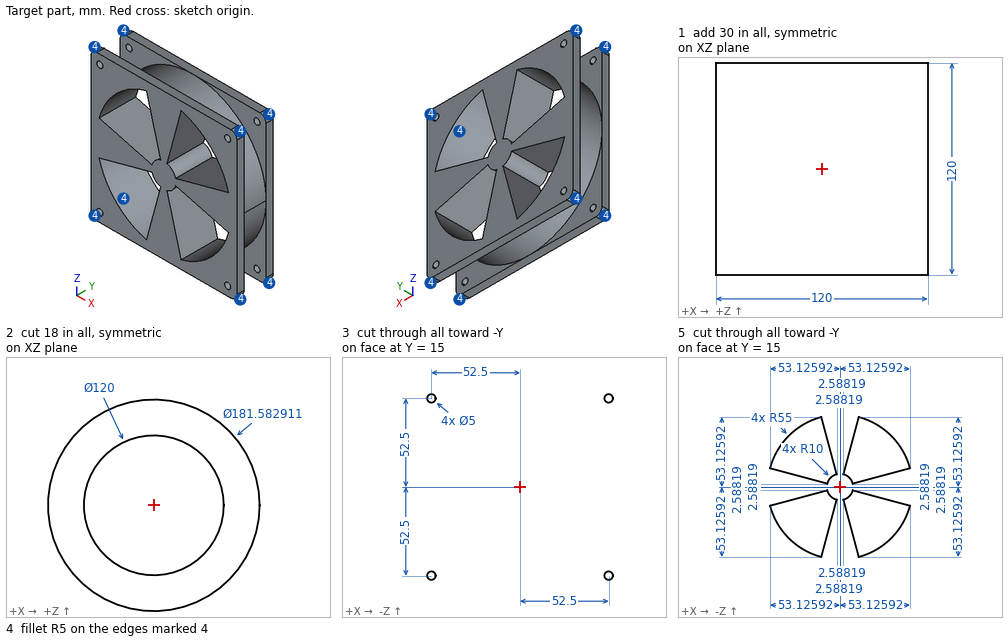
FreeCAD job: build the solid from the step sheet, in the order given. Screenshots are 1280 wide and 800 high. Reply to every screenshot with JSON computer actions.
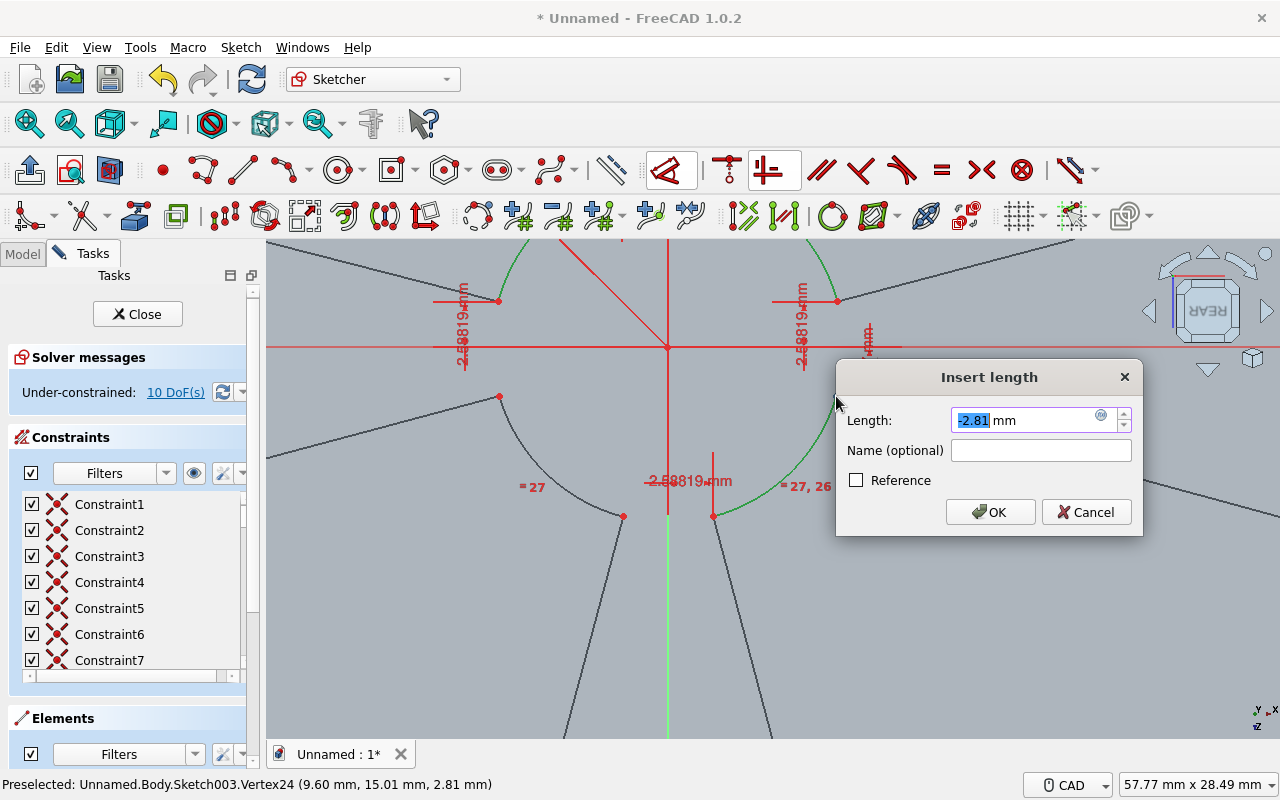
{"action": "type", "text": "-2.58819"}
{"action": "key", "text": "Return"}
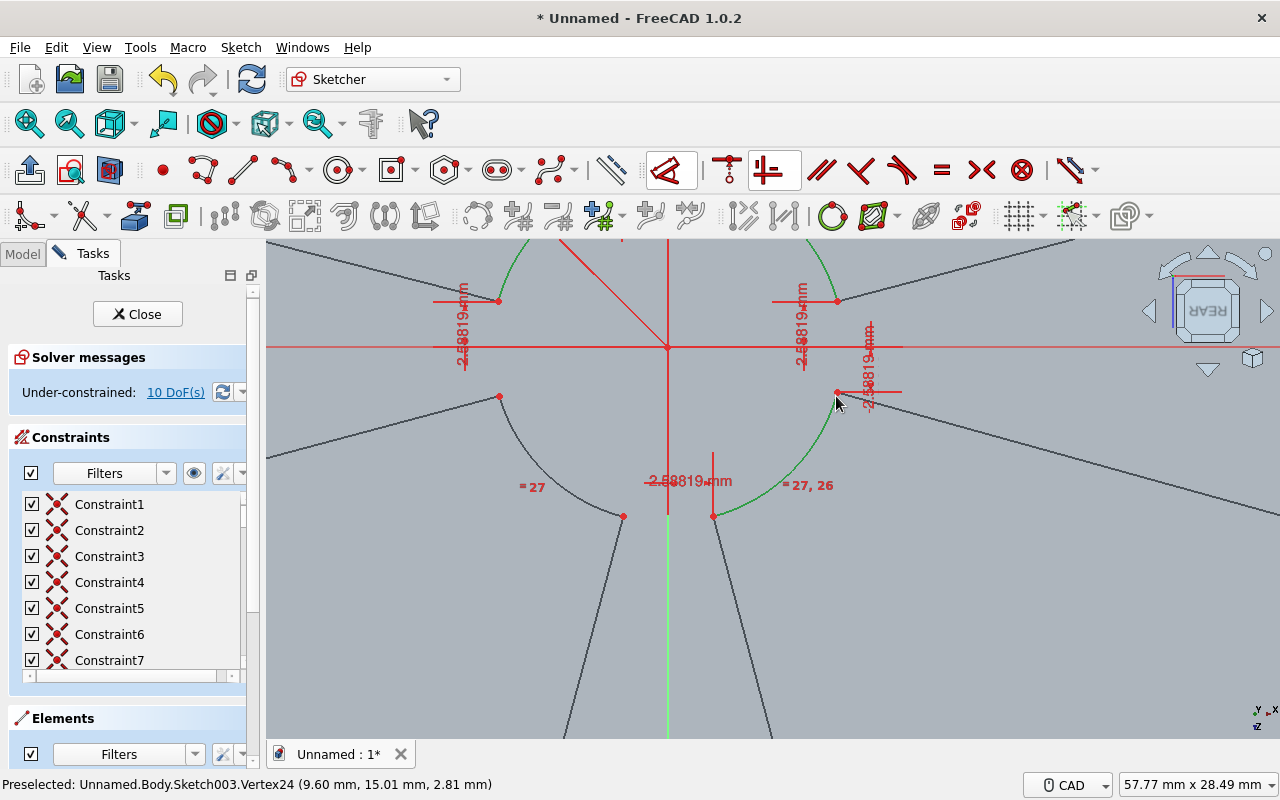
{"action": "left_click", "coordinate": [623, 517]}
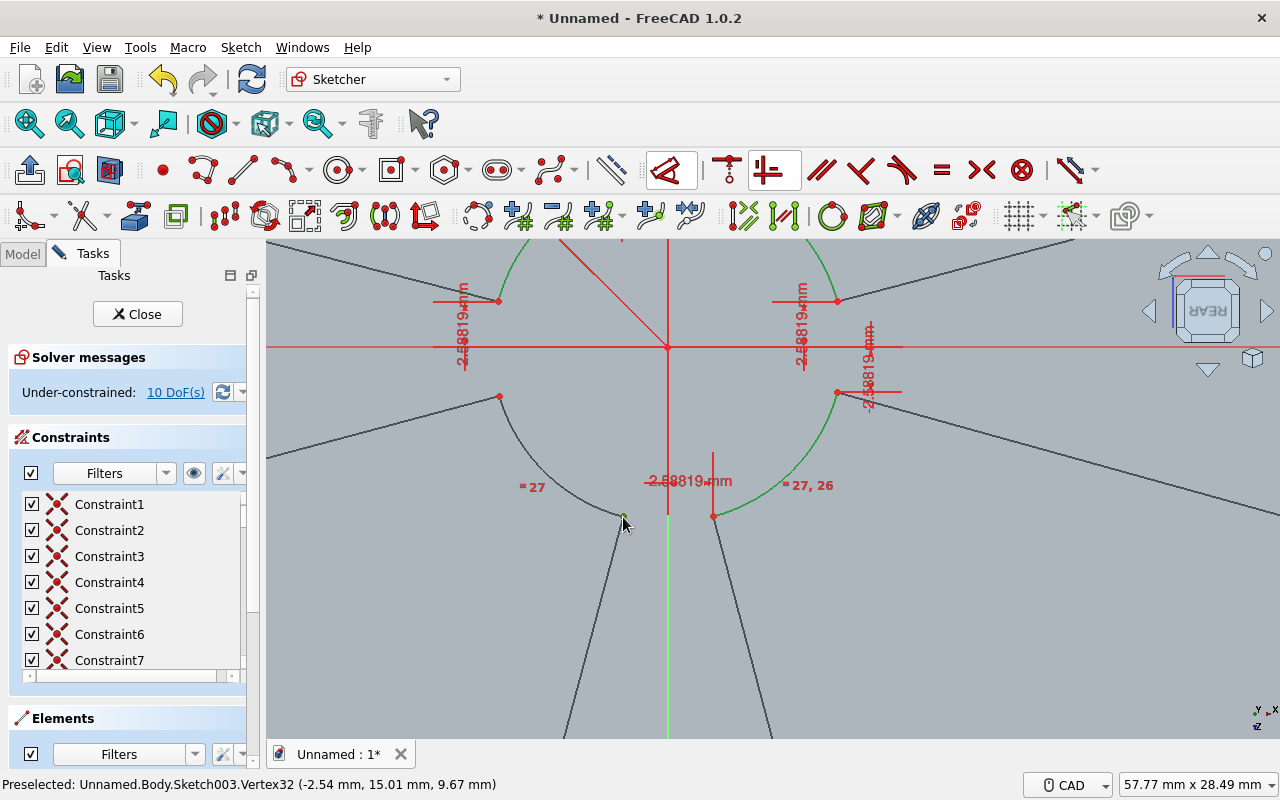
{"action": "key", "text": "l"}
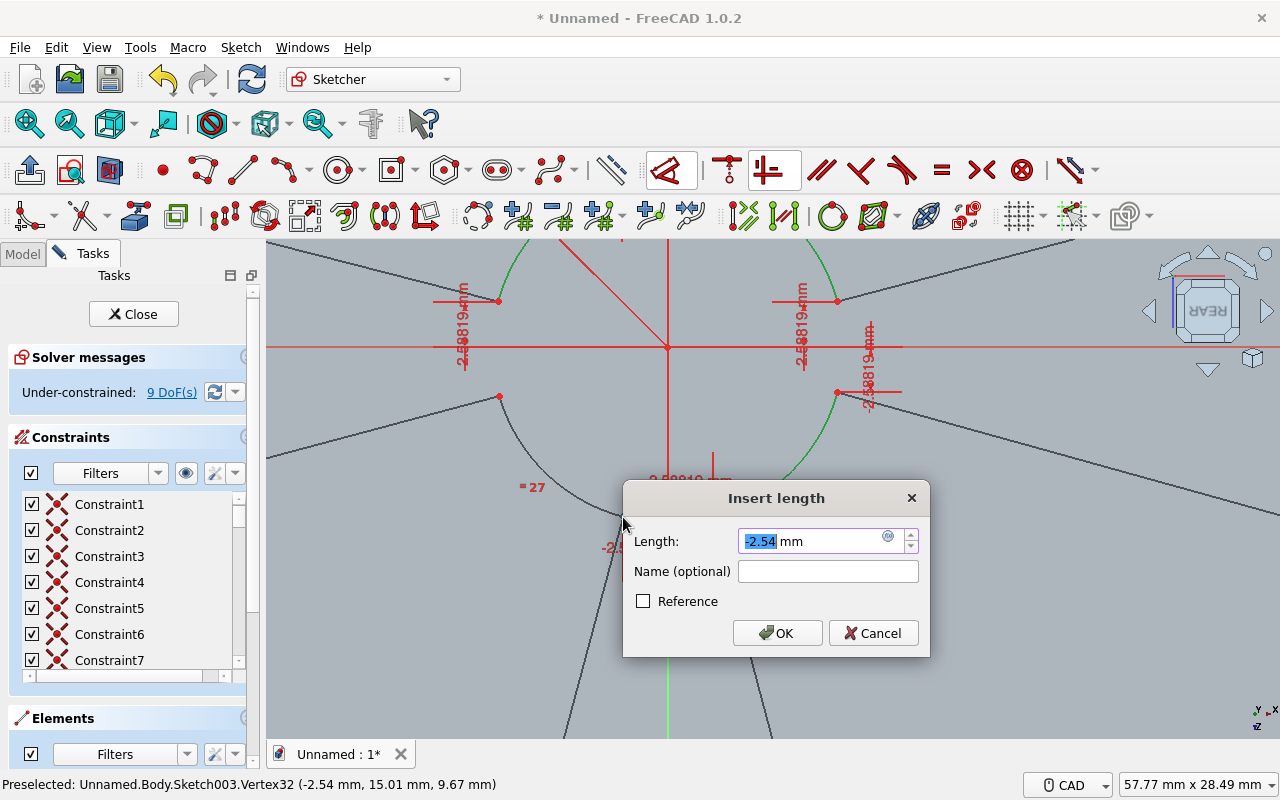
{"action": "type", "text": "-2.58819"}
{"action": "key", "text": "Return"}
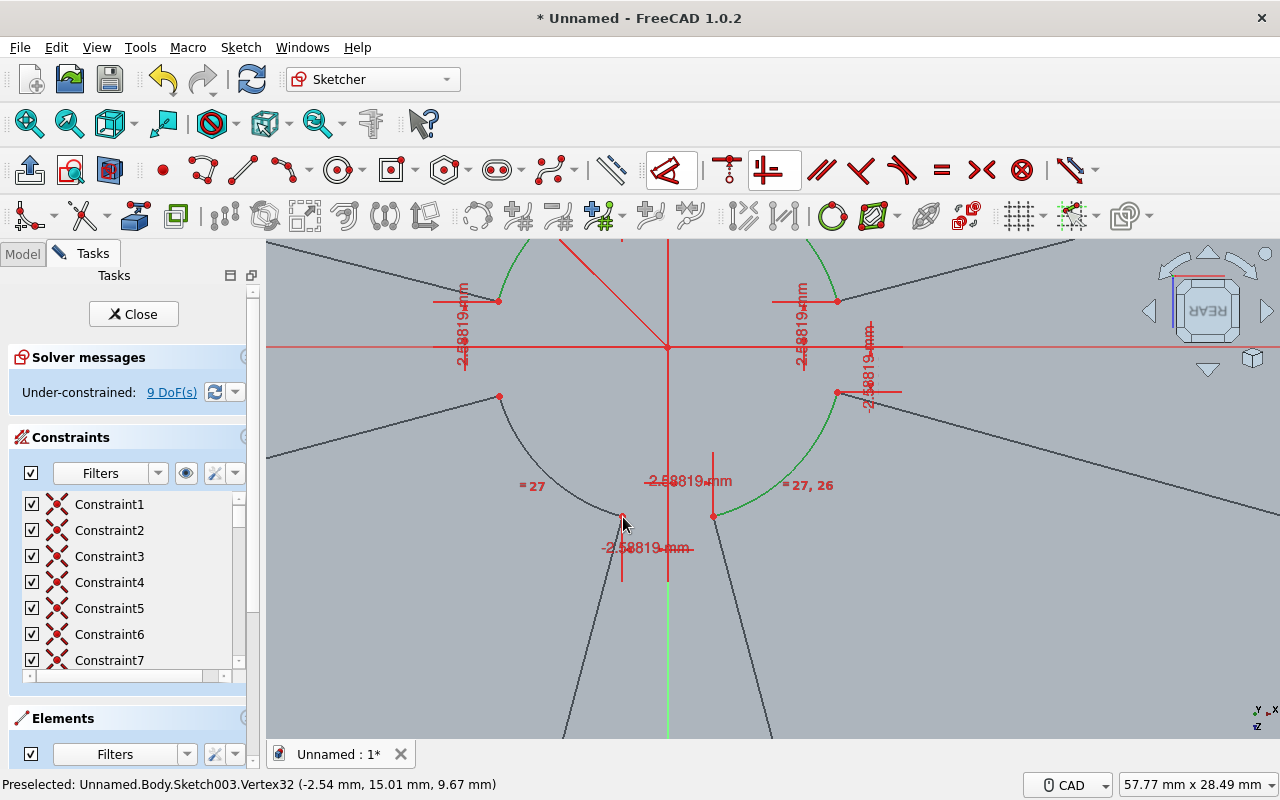
{"action": "left_click", "coordinate": [499, 396]}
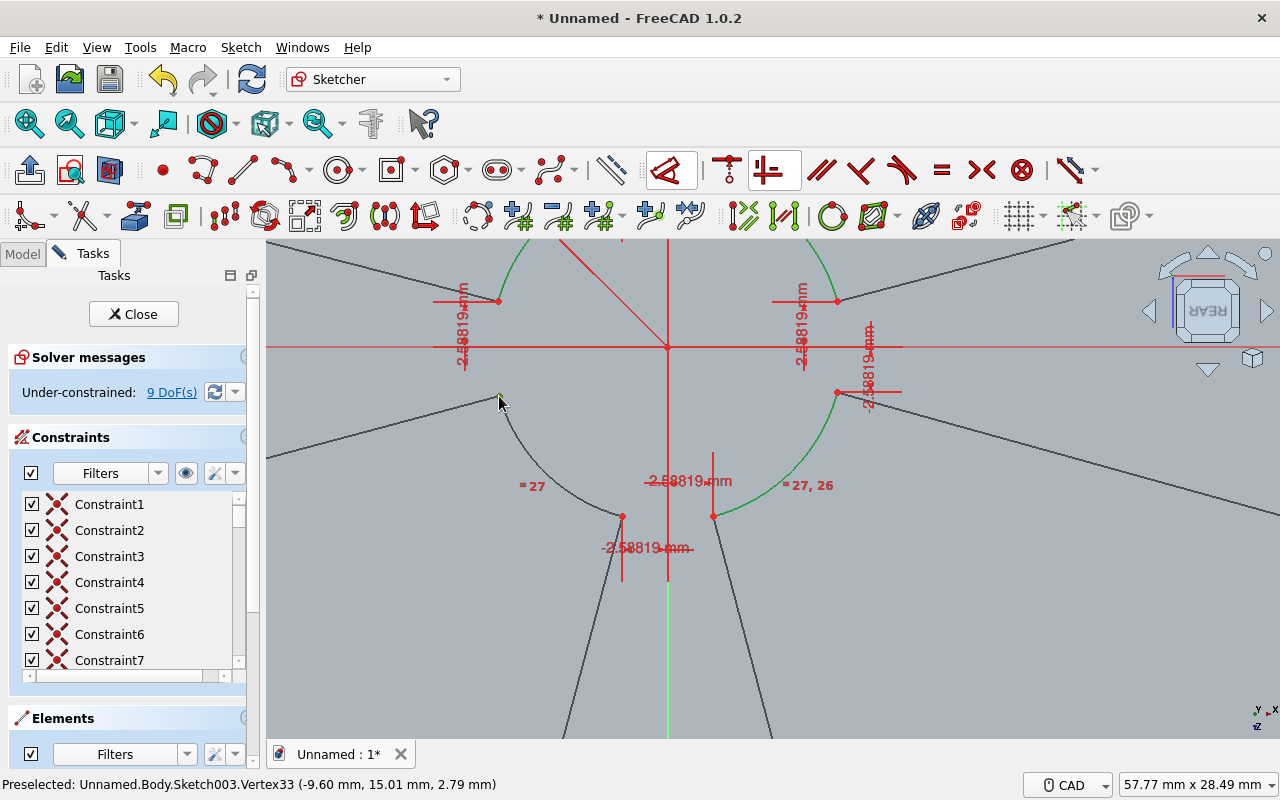
{"action": "left_click", "coordinate": [692, 170]}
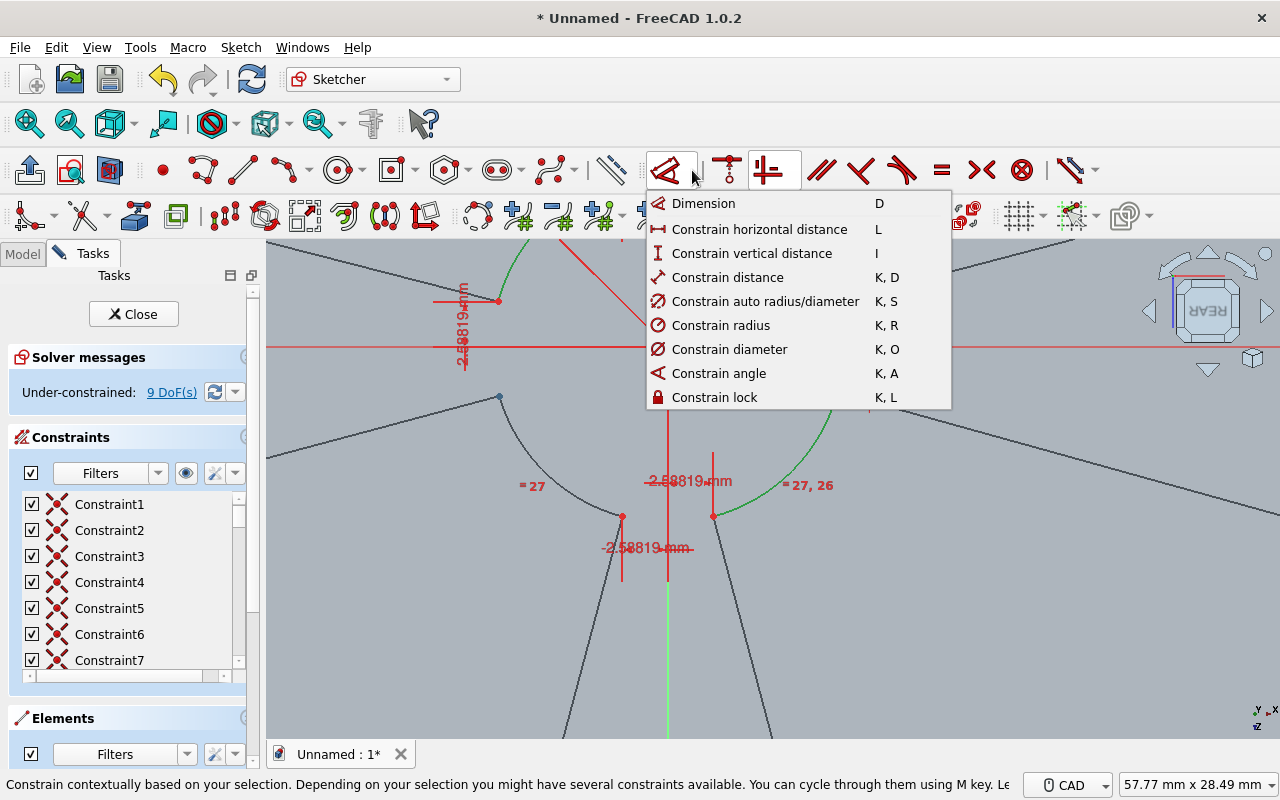
{"action": "left_click", "coordinate": [799, 253]}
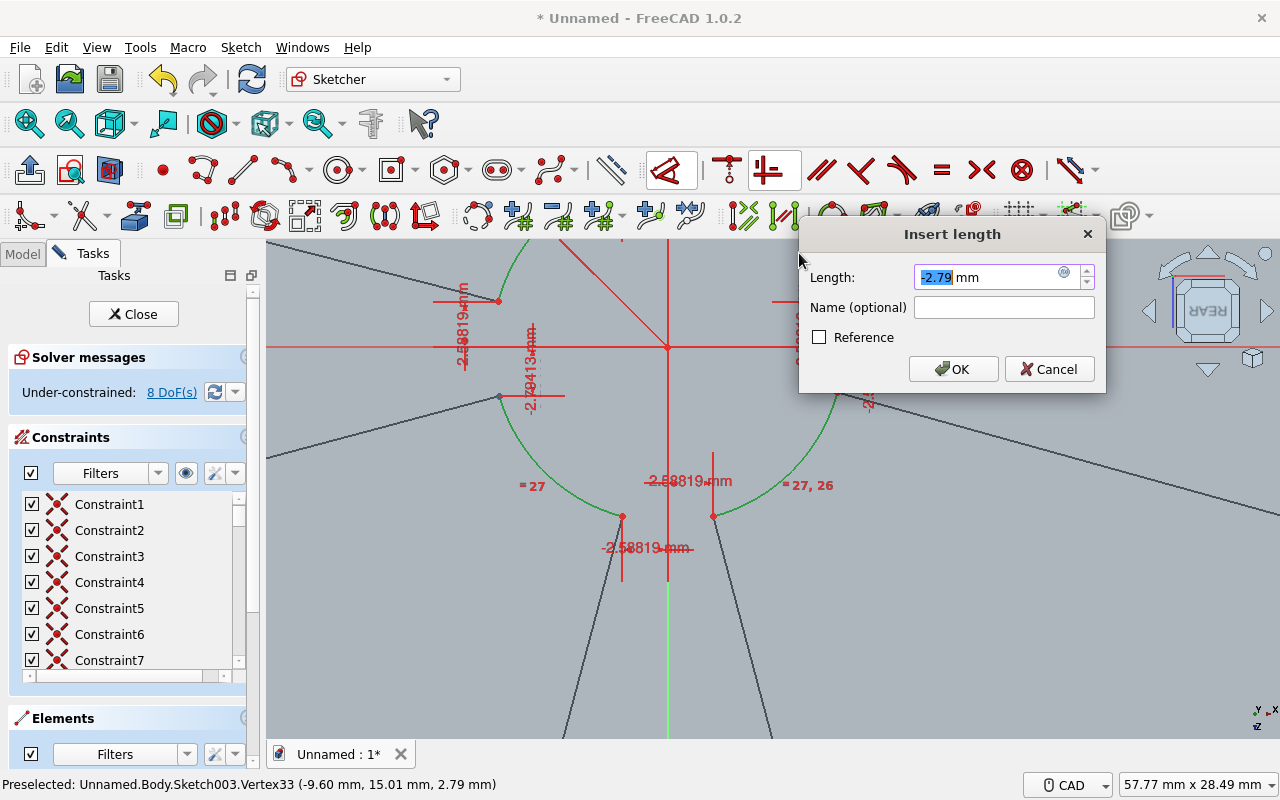
{"action": "type", "text": "-2.58819"}
{"action": "key", "text": "Return"}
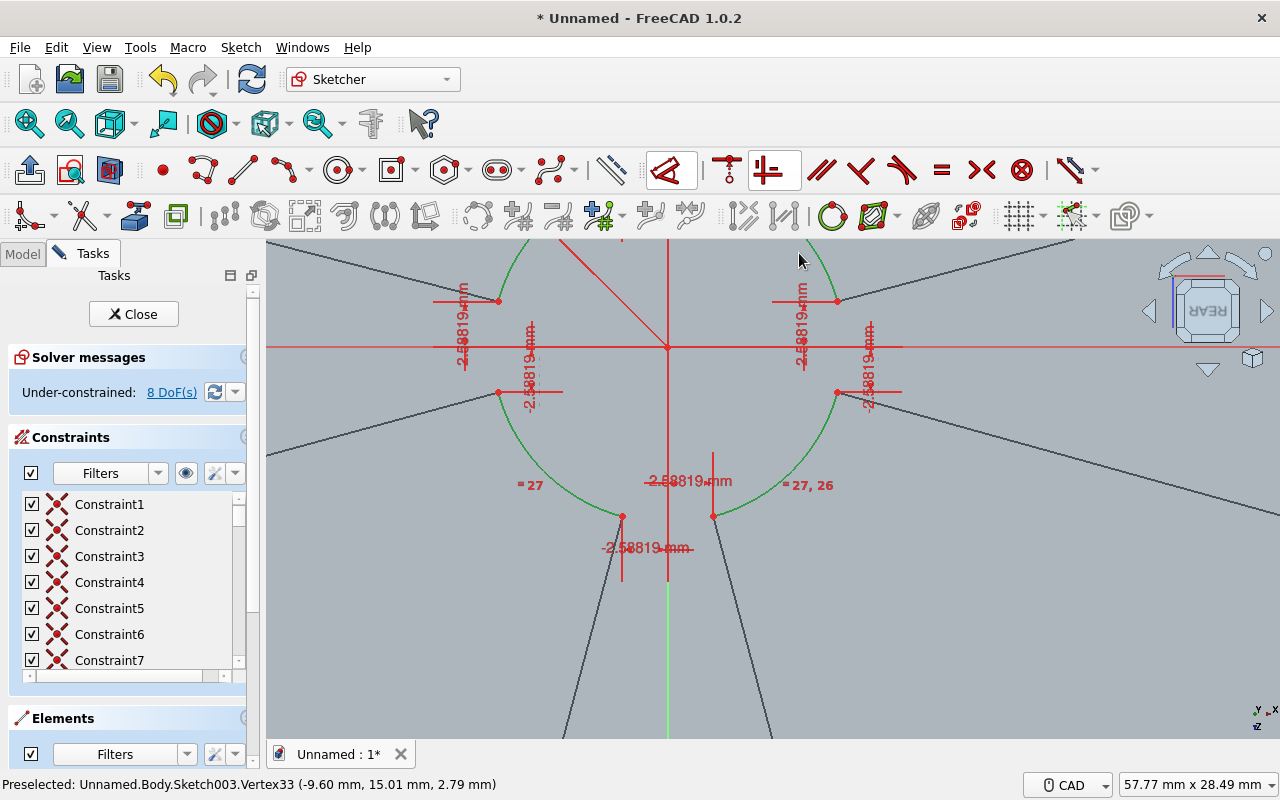
{"action": "scroll", "coordinate": [712, 517], "scroll_direction": "down", "scroll_amount": 9}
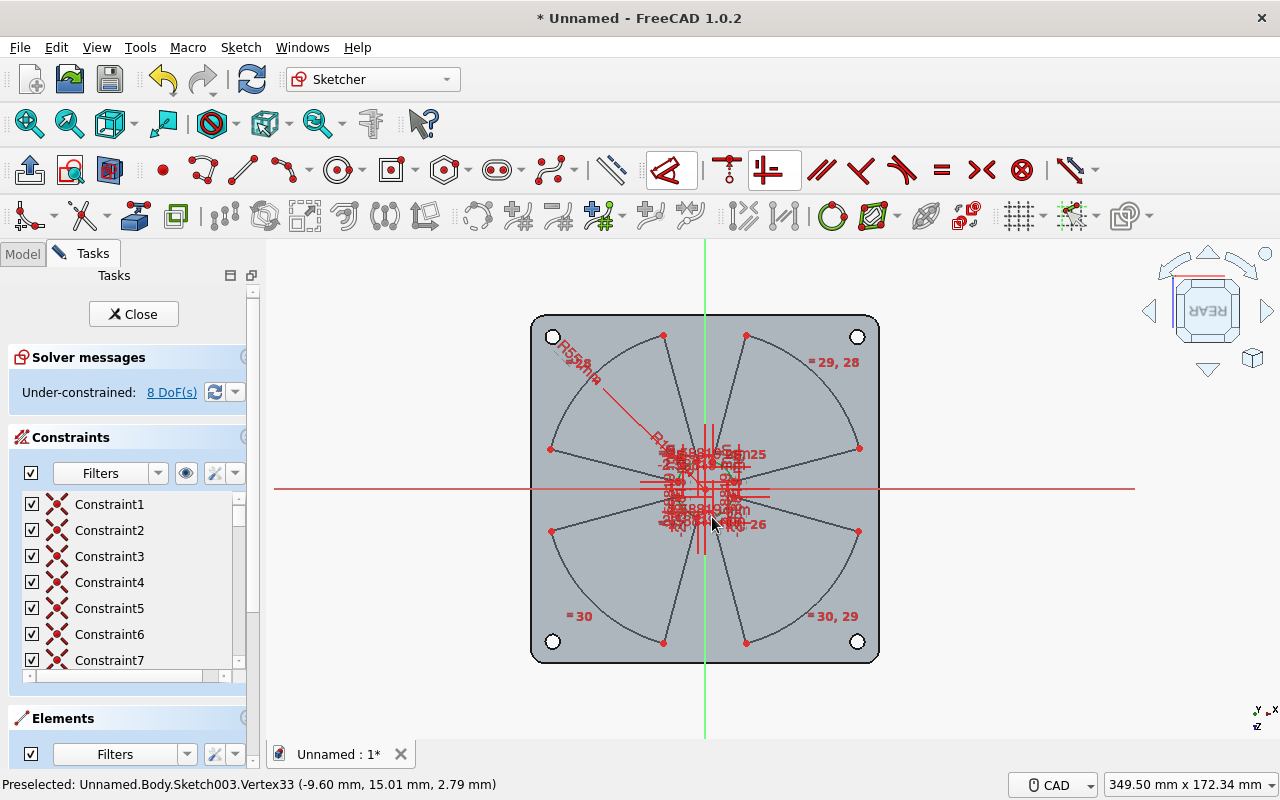
{"action": "left_click", "coordinate": [663, 335]}